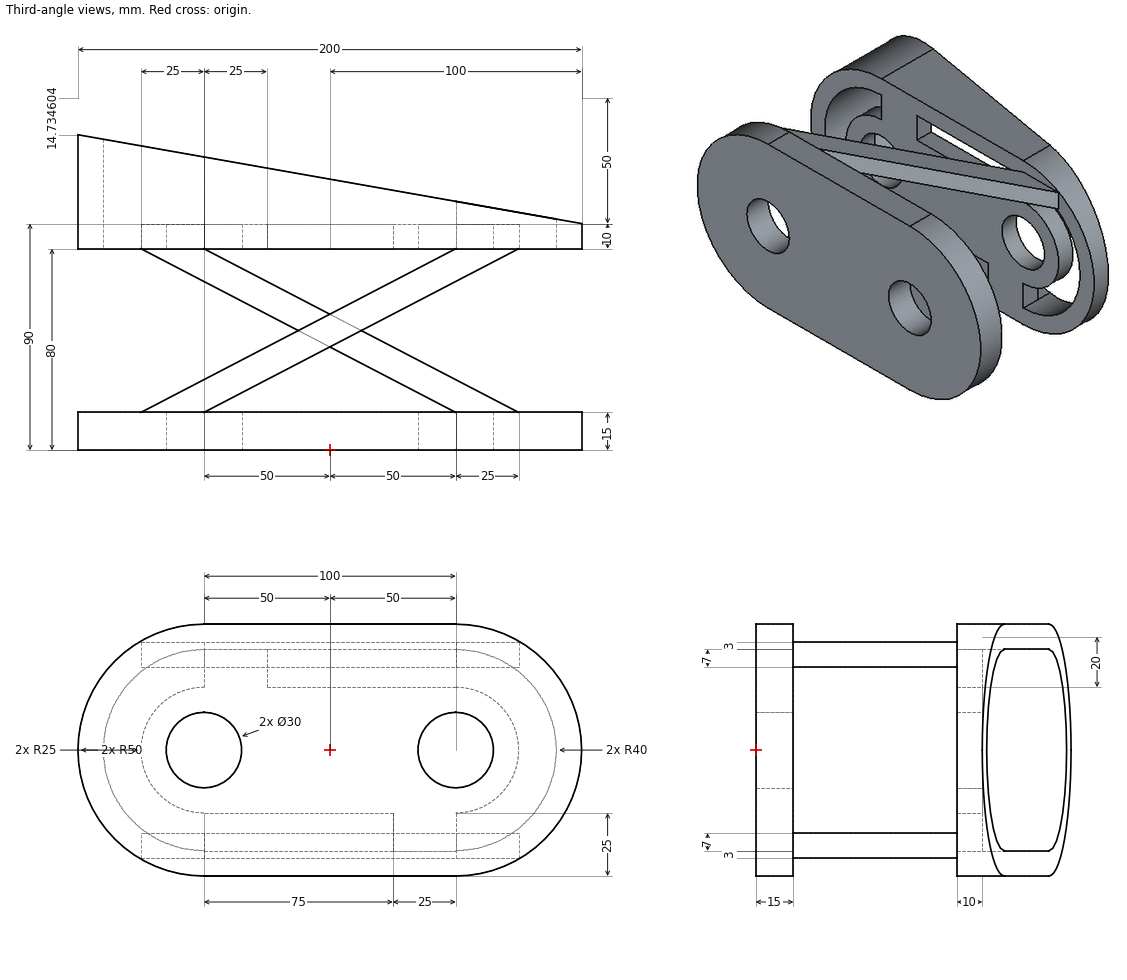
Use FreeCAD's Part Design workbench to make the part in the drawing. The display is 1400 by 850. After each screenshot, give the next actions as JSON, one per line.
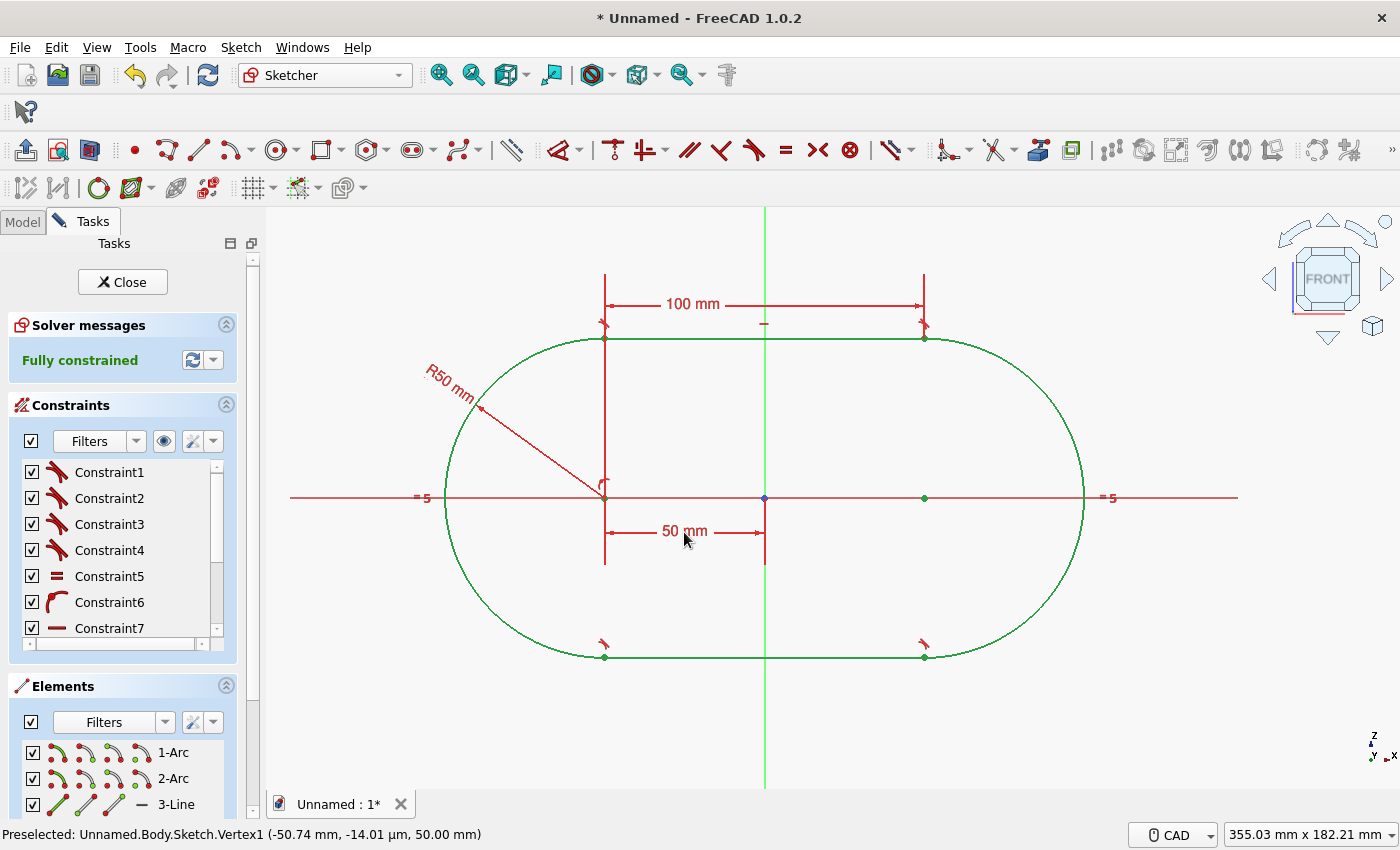
{"action": "left_click", "coordinate": [123, 282]}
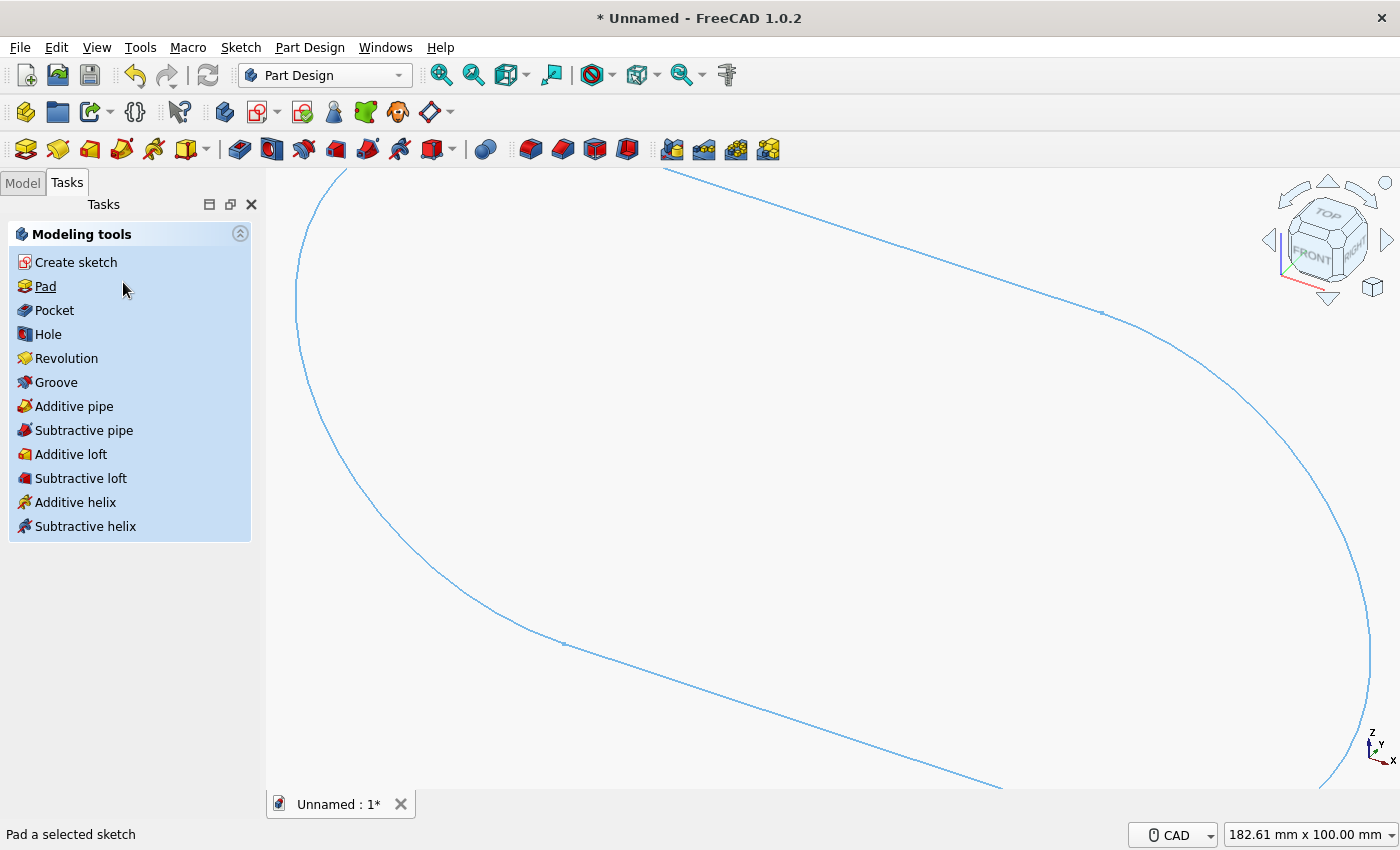
{"action": "left_click", "coordinate": [26, 150]}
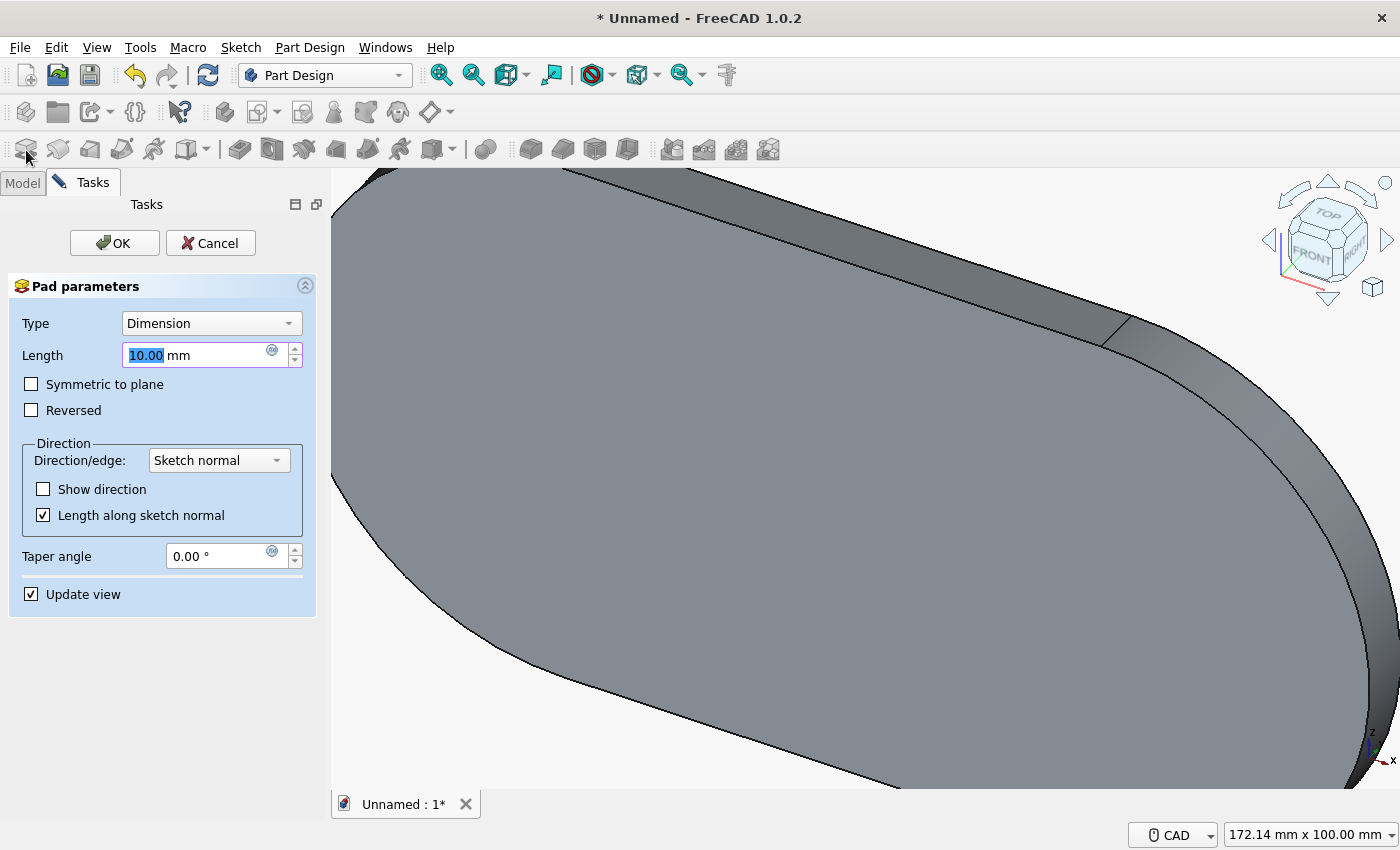
{"action": "type", "text": "15"}
{"action": "key", "text": "Tab"}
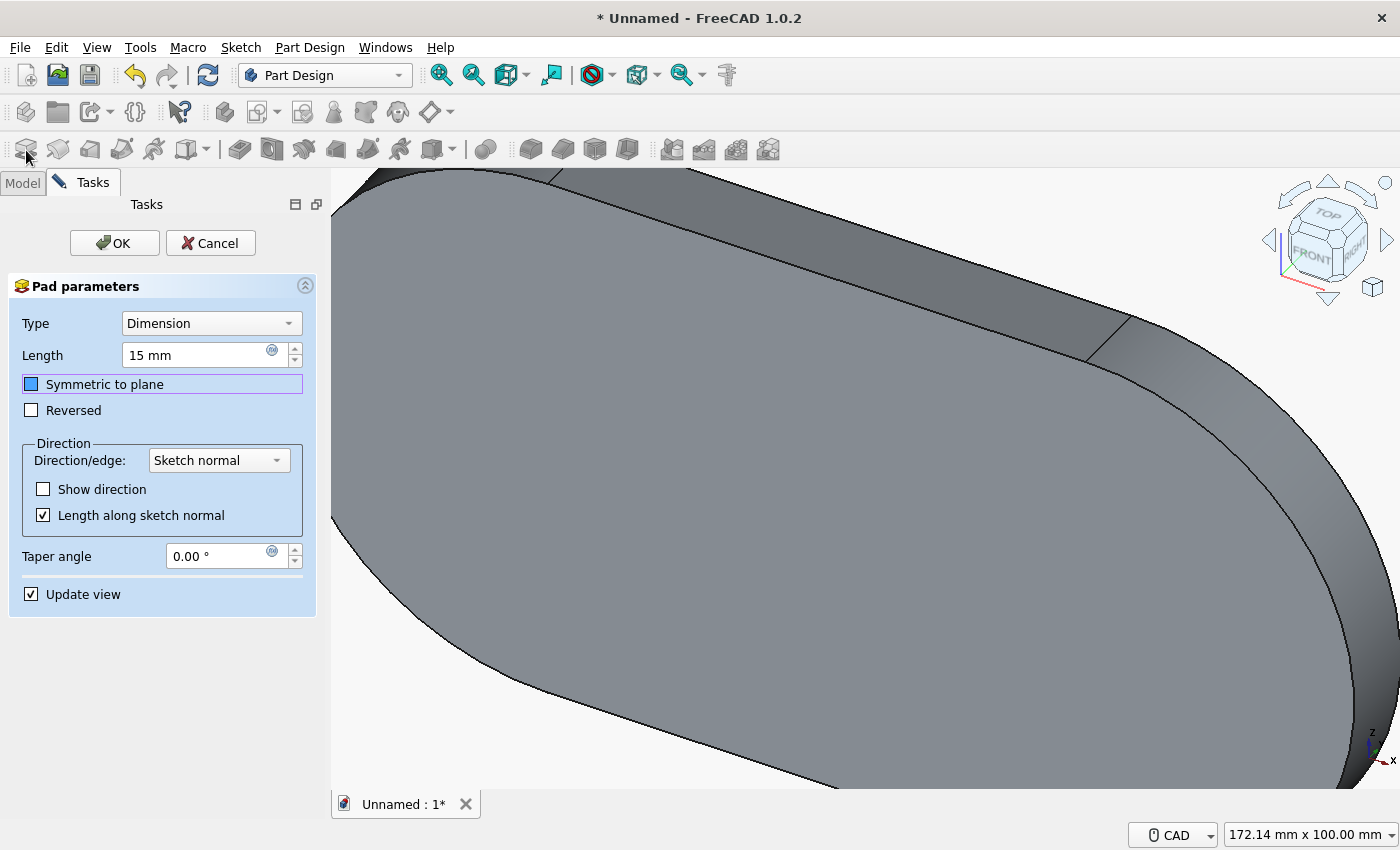
{"action": "left_click", "coordinate": [30, 410]}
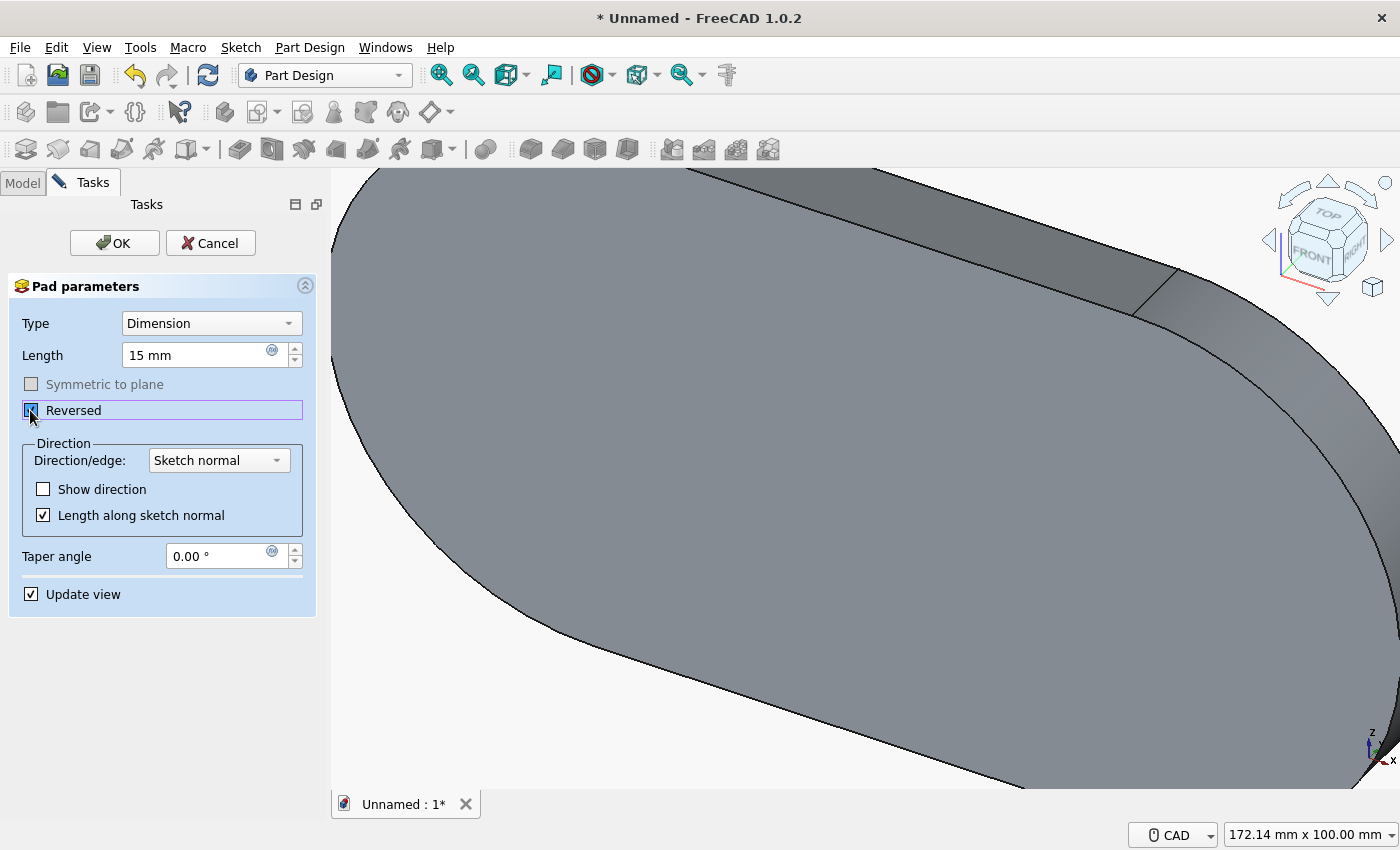
{"action": "left_click", "coordinate": [115, 243]}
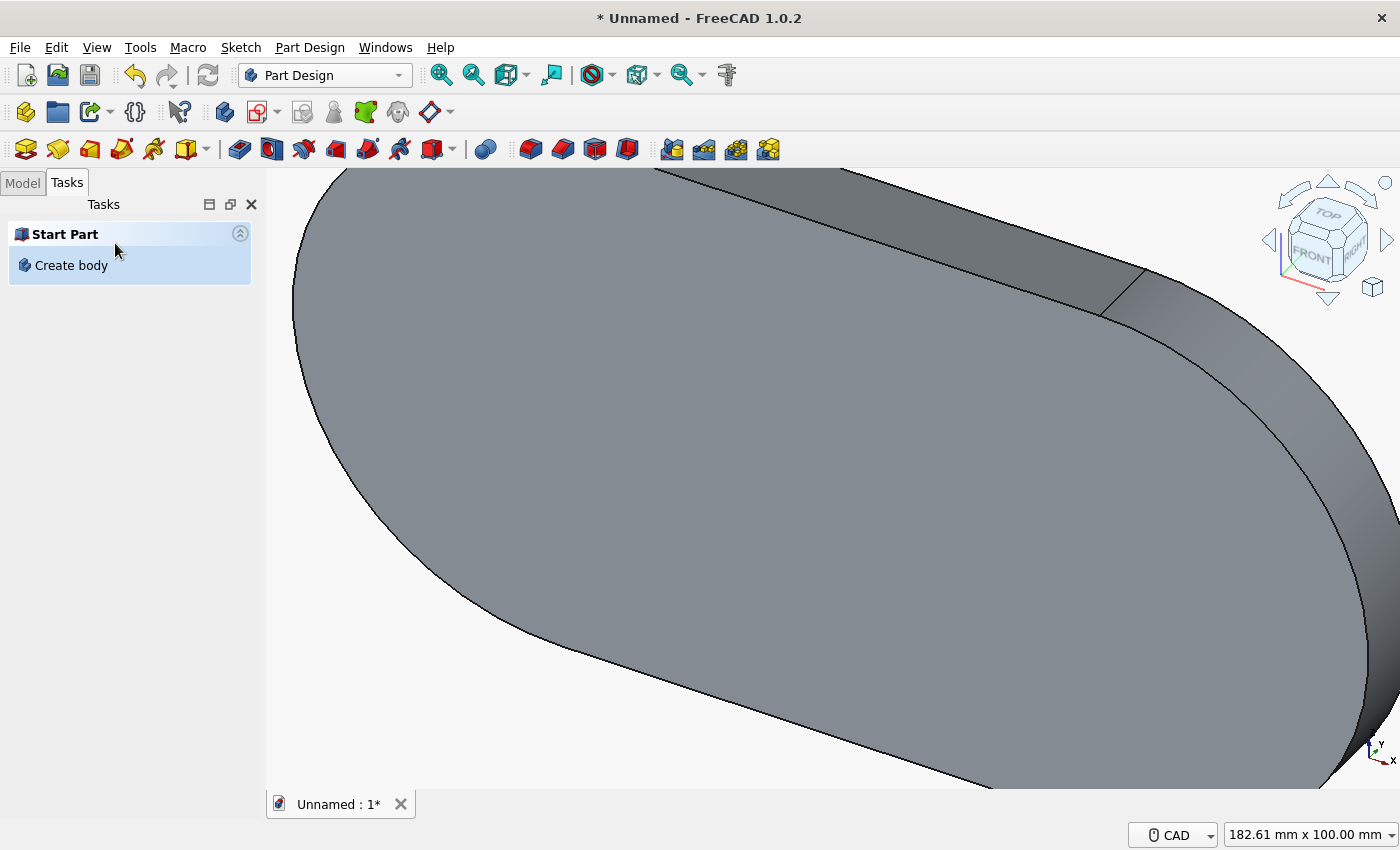
{"action": "left_click", "coordinate": [442, 76]}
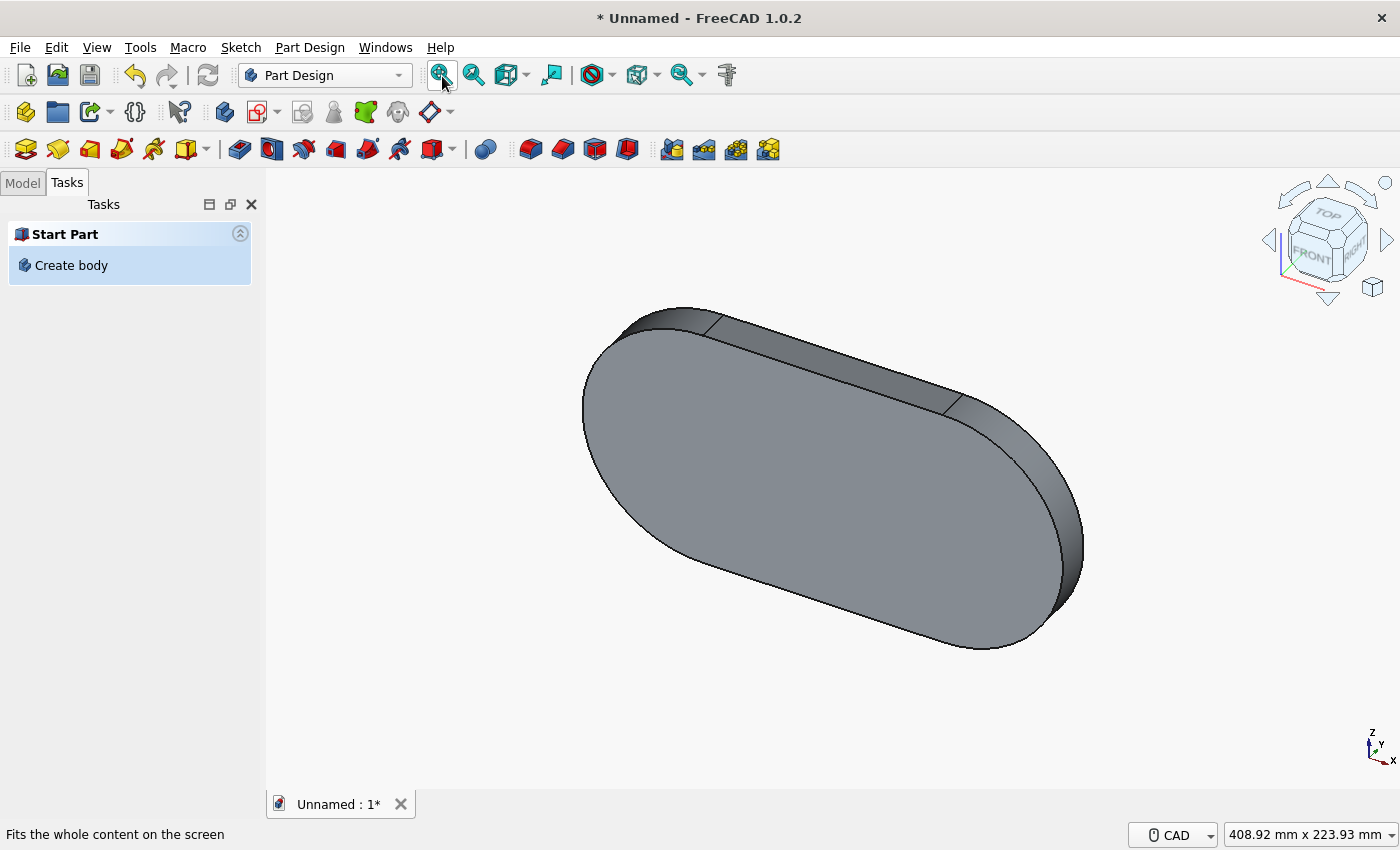
{"action": "left_click", "coordinate": [226, 112]}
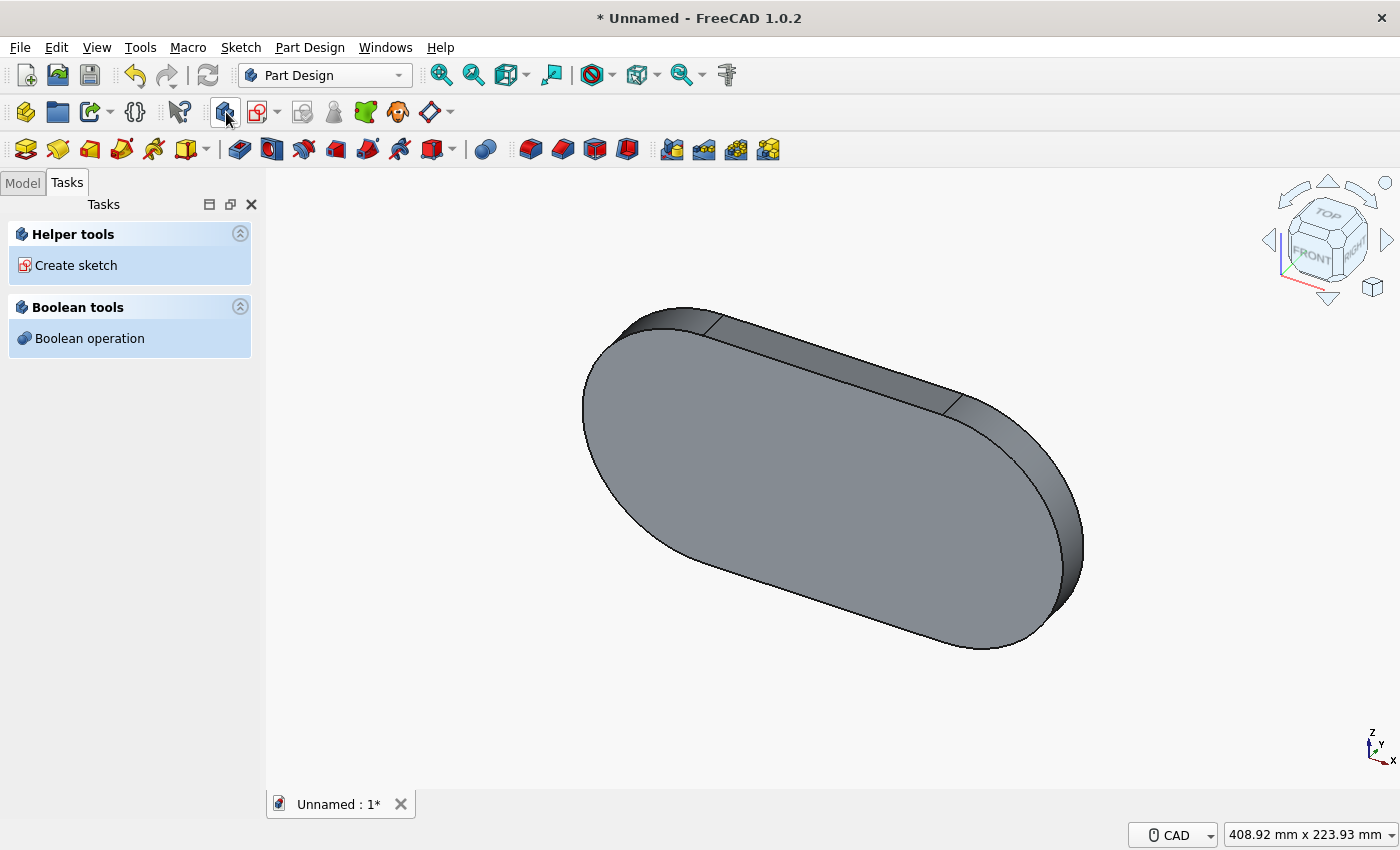
{"action": "left_click", "coordinate": [23, 182]}